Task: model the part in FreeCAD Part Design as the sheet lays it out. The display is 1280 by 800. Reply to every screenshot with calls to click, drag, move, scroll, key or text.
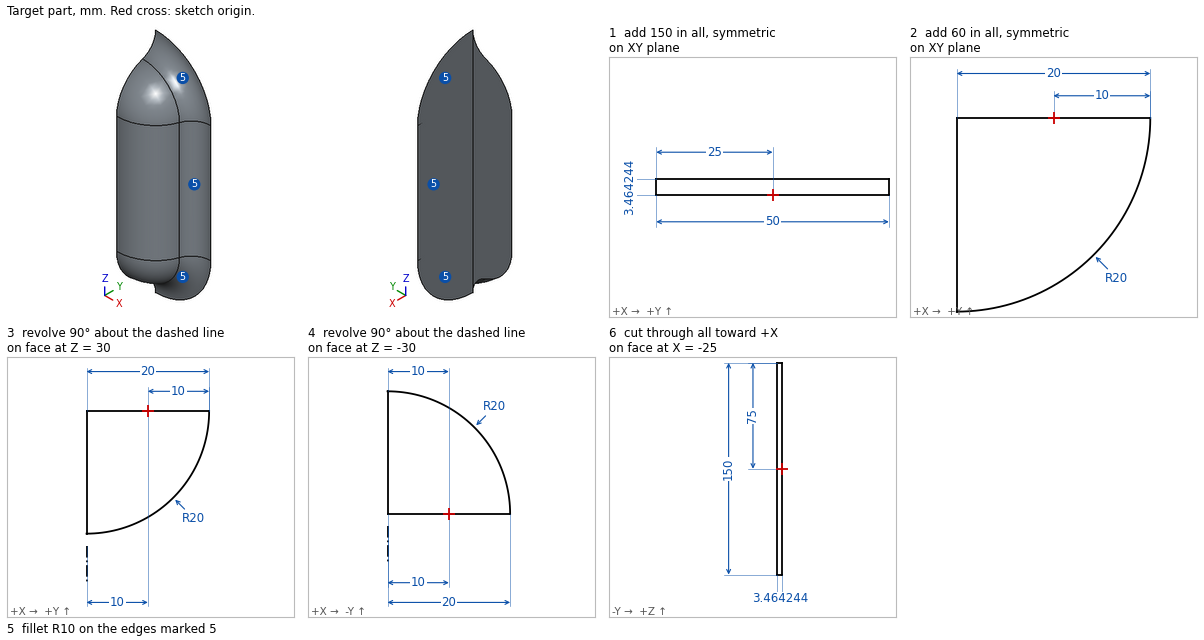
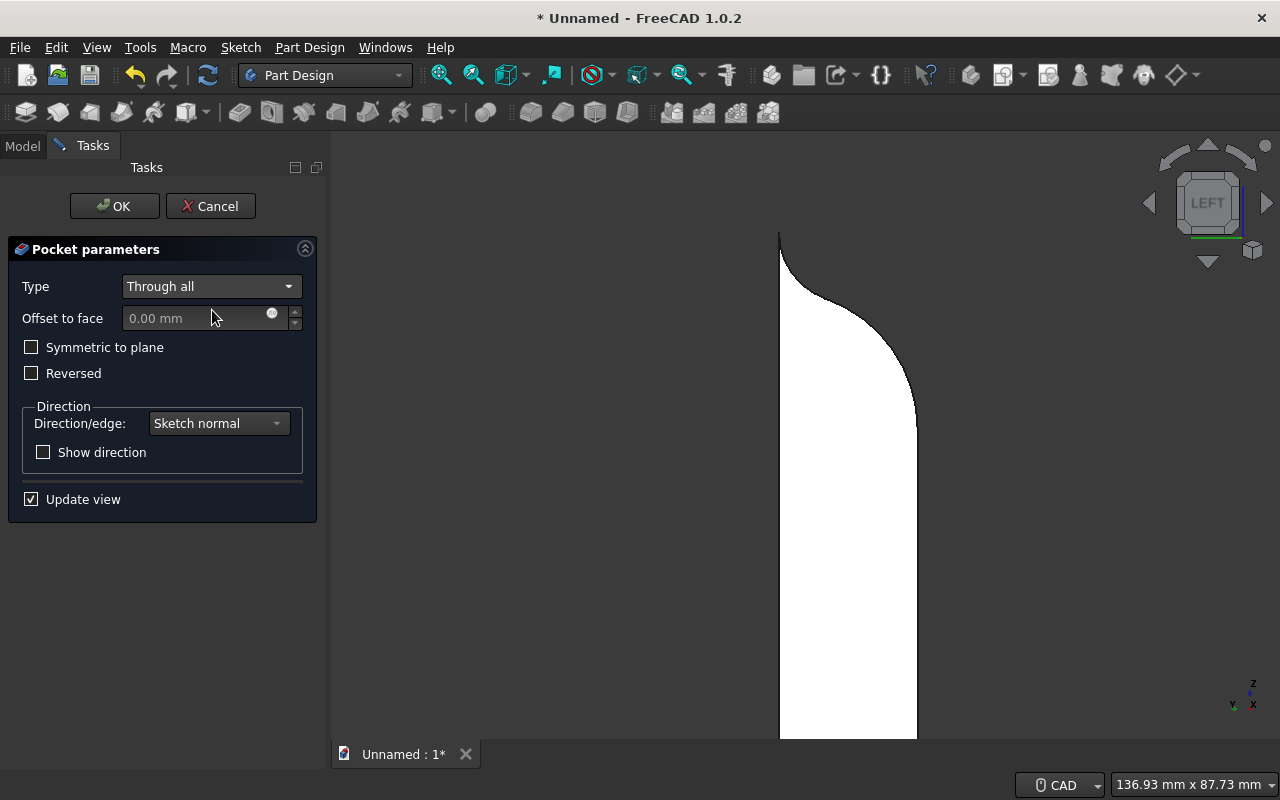
click(115, 206)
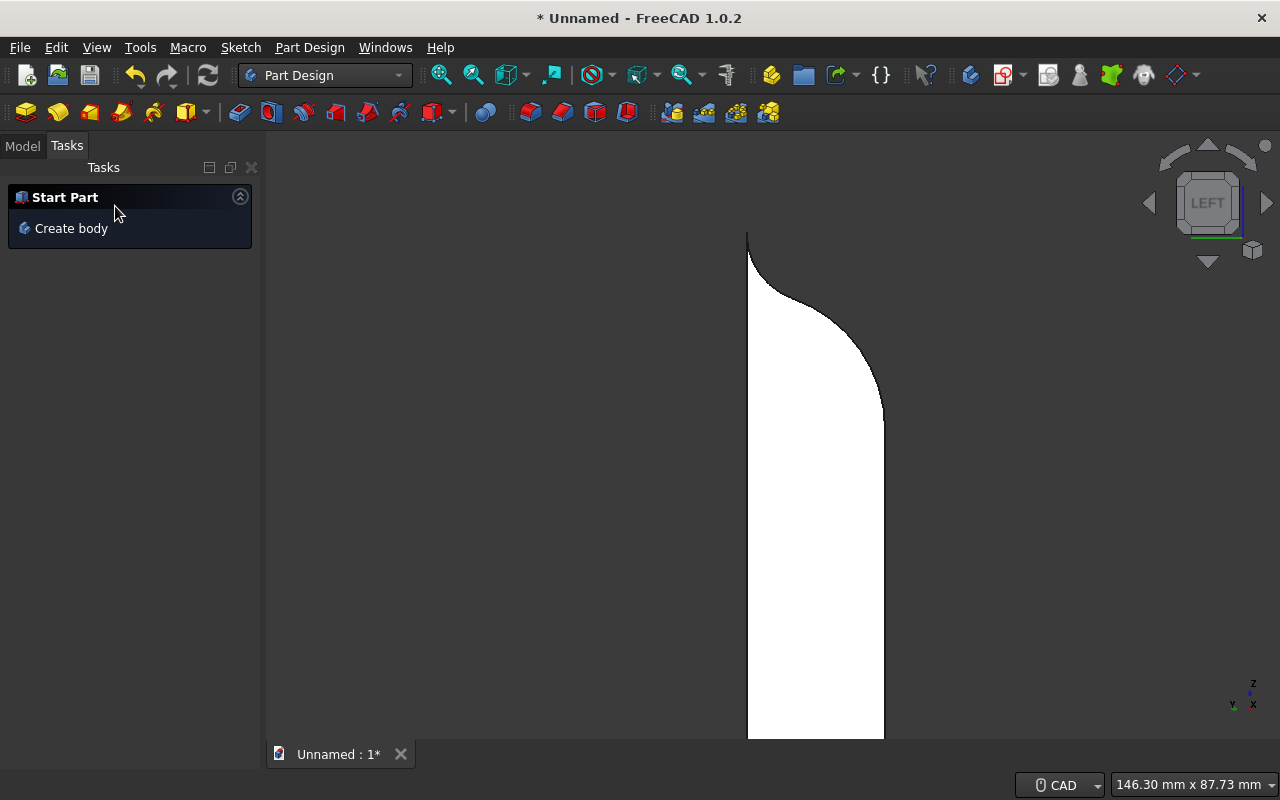
key(0)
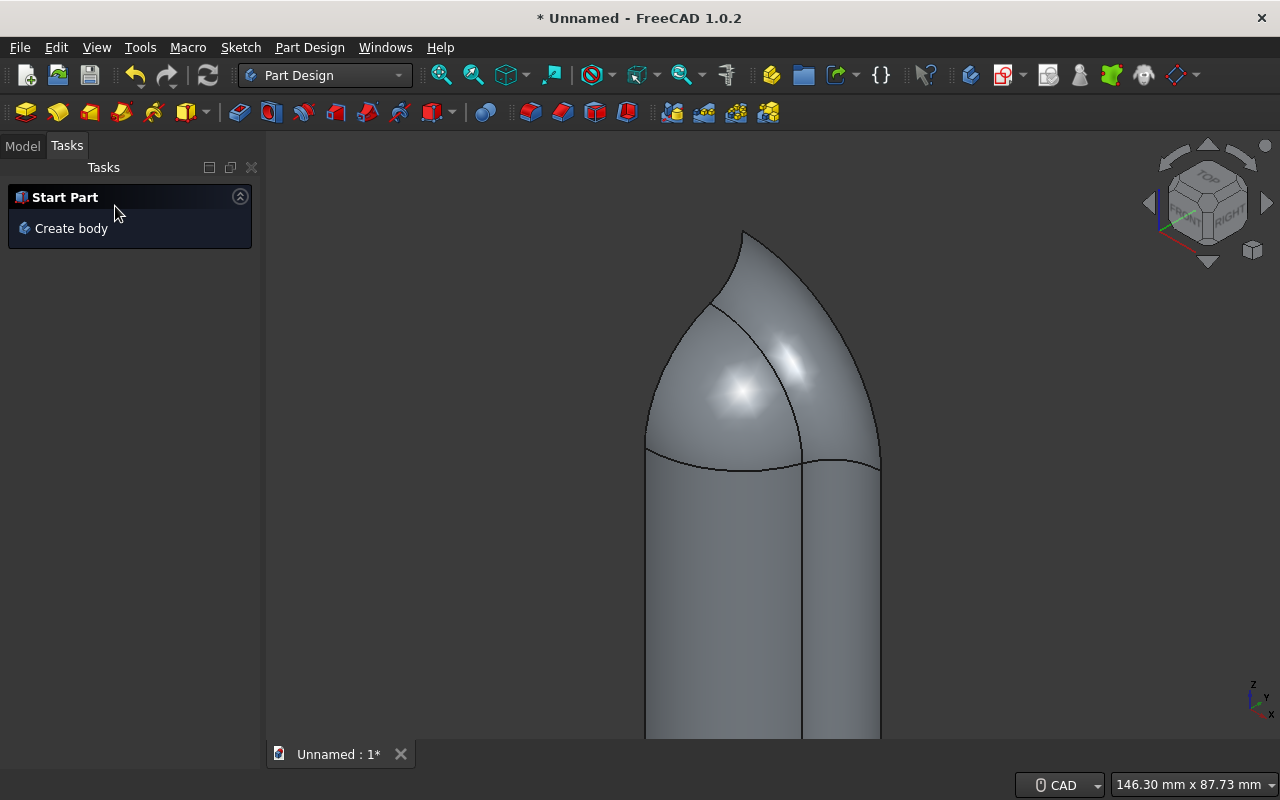
click(442, 76)